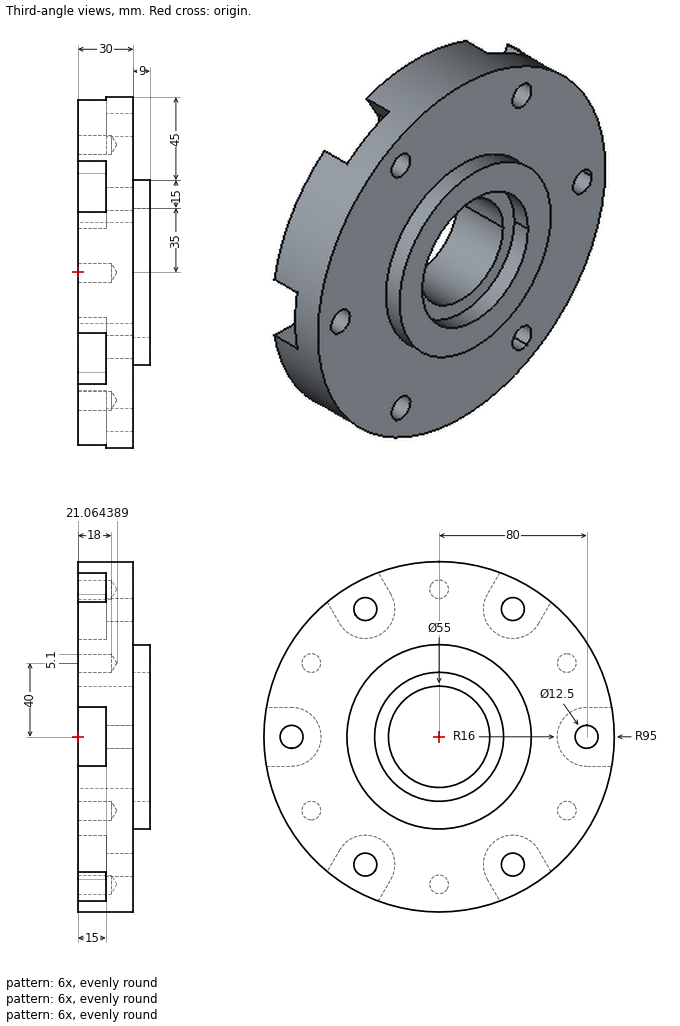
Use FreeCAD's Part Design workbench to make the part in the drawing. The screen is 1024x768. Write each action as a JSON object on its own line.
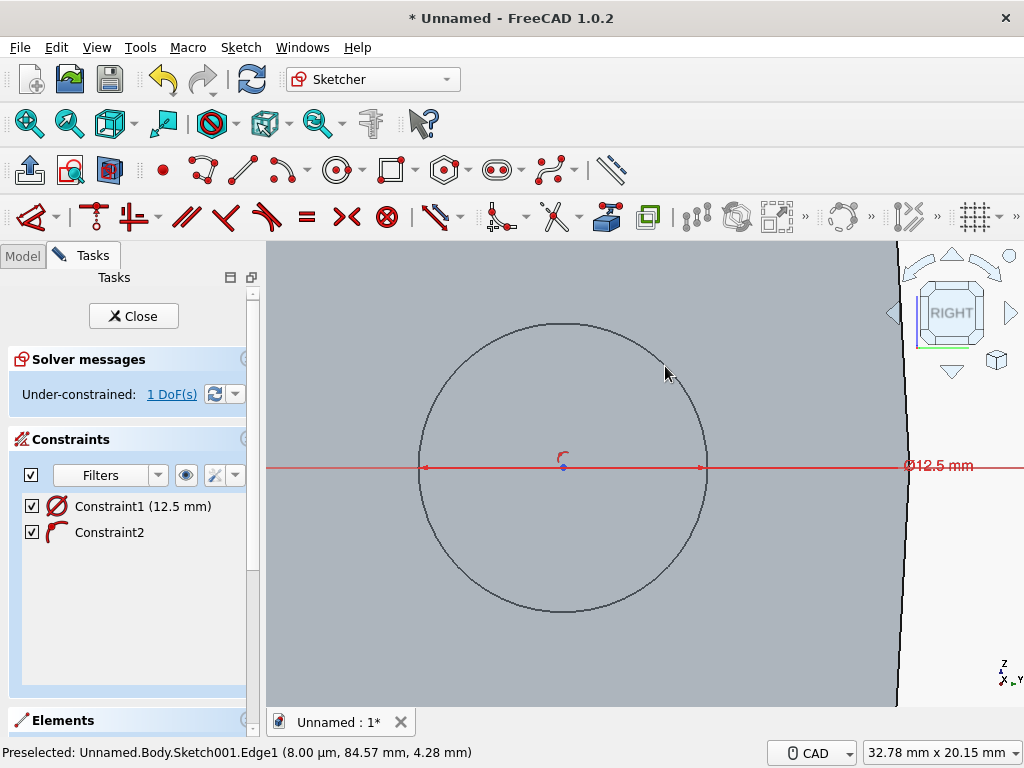
{"action": "key", "text": "d"}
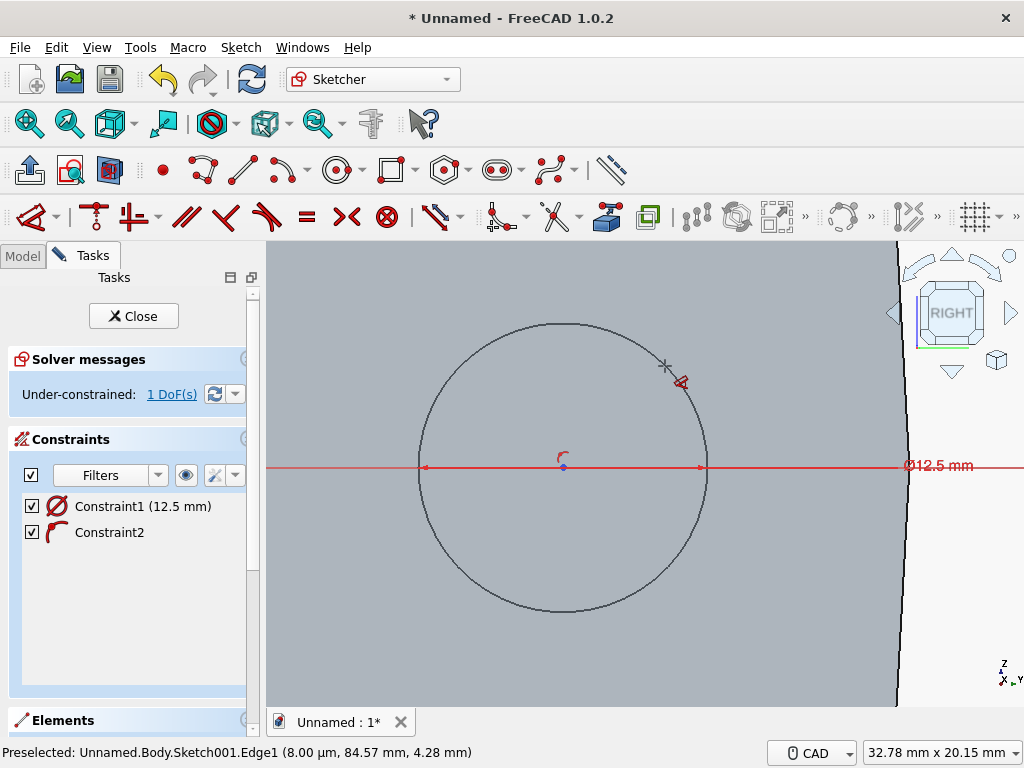
{"action": "left_click", "coordinate": [563, 468]}
{"action": "left_click", "coordinate": [367, 502]}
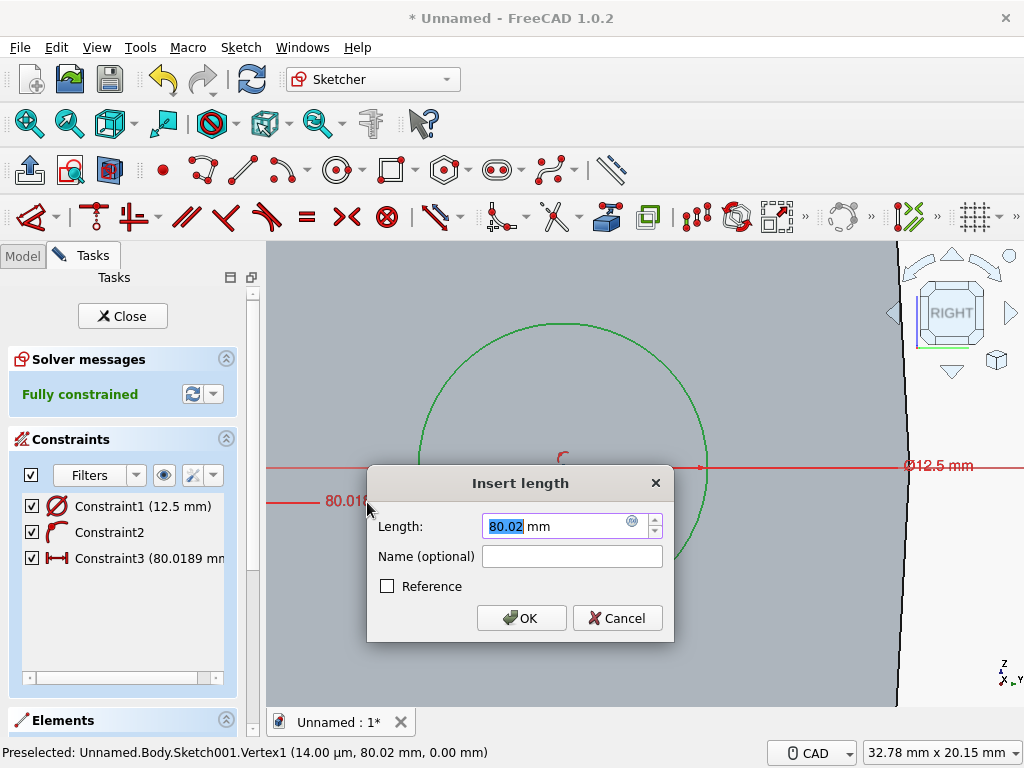
{"action": "type", "text": "80"}
{"action": "key", "text": "Return"}
{"action": "key", "text": "Escape"}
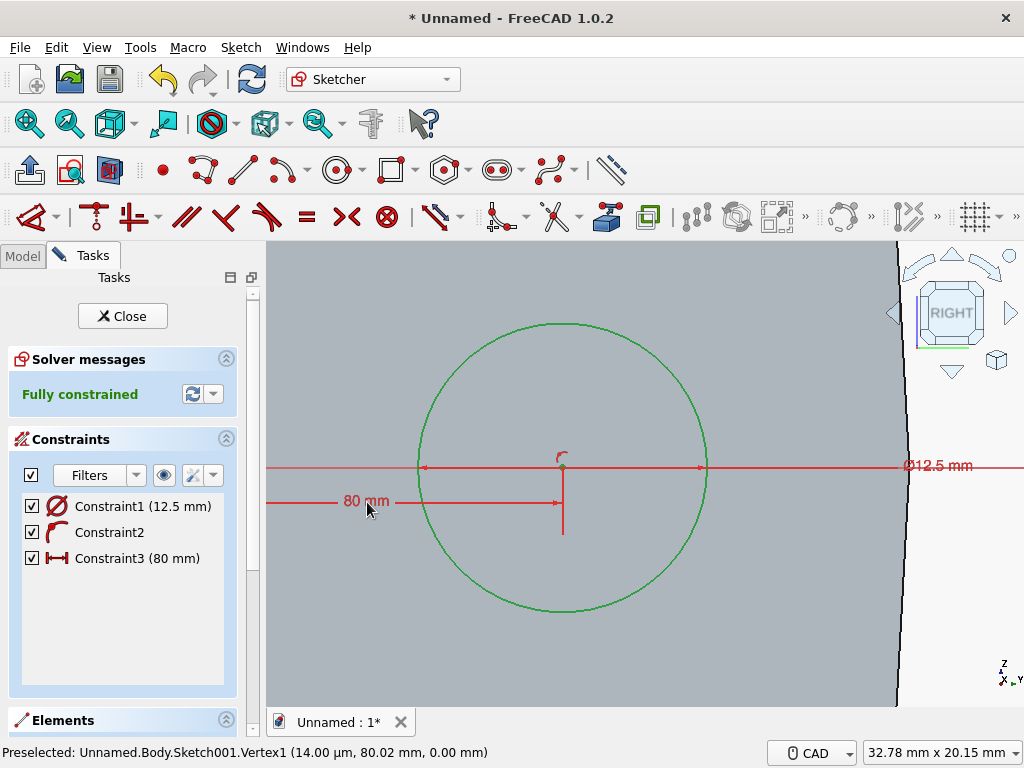
{"action": "left_click", "coordinate": [123, 316]}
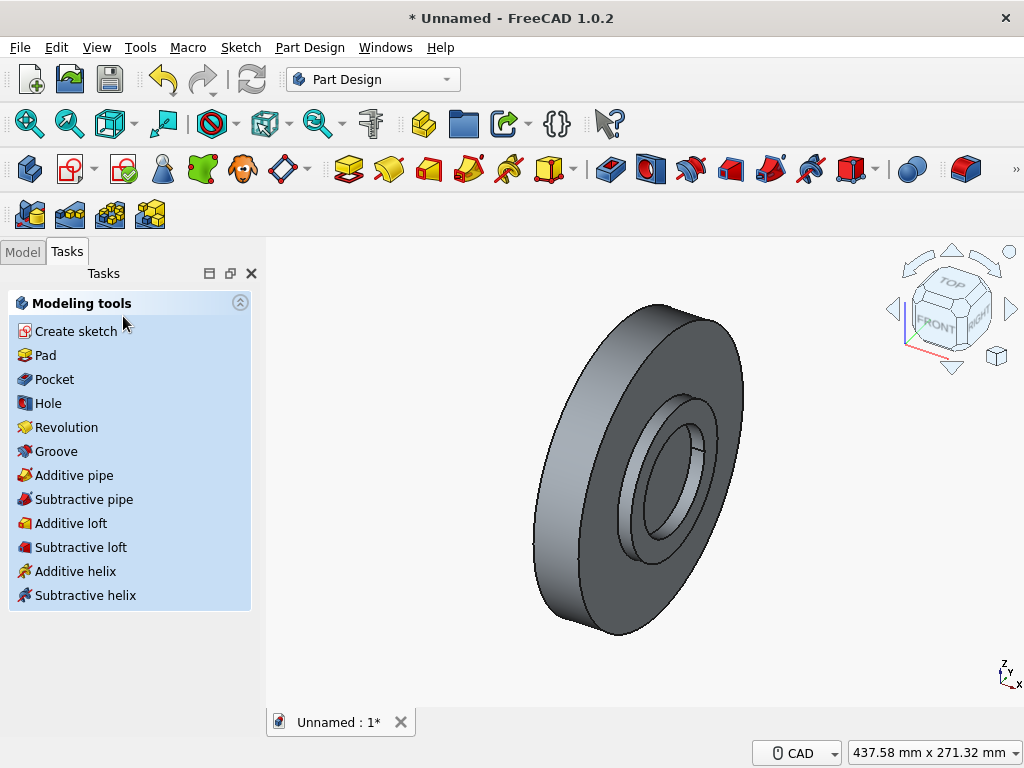
{"action": "left_click", "coordinate": [612, 170]}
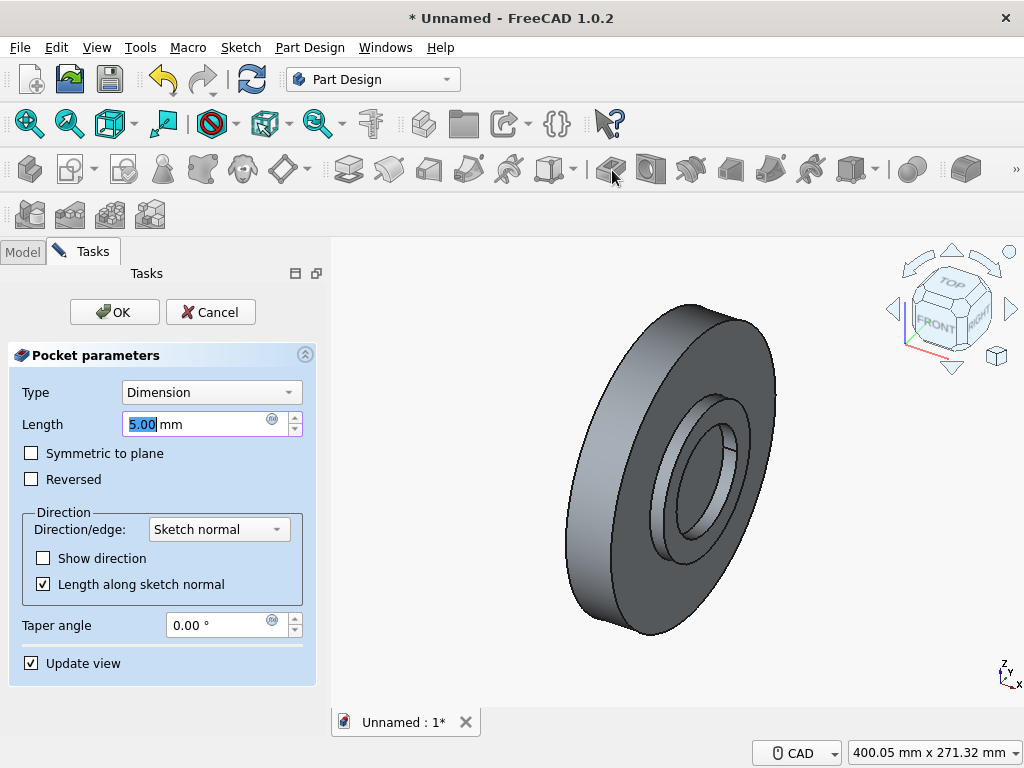
{"action": "left_click", "coordinate": [212, 392]}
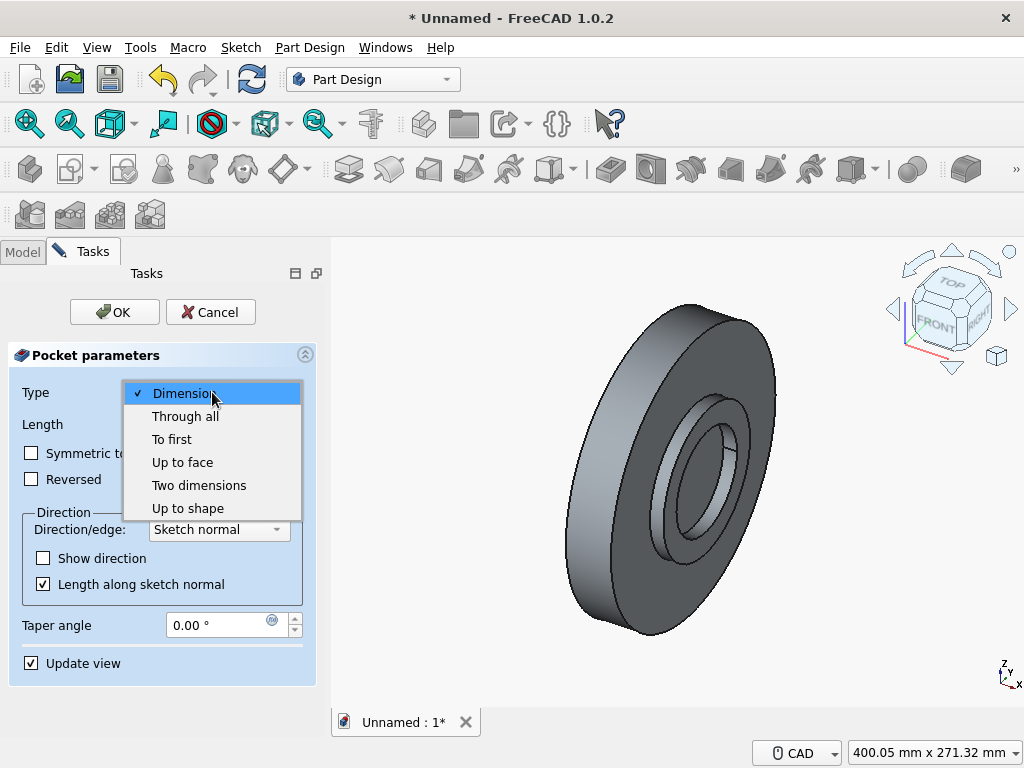
{"action": "left_click", "coordinate": [212, 416]}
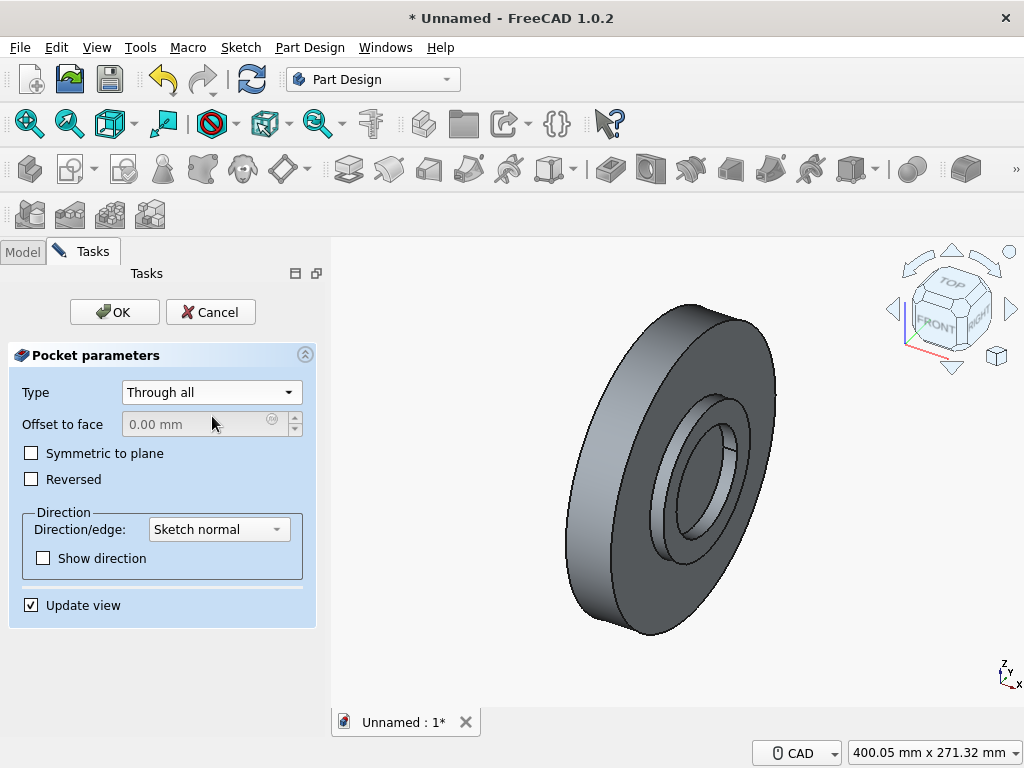
{"action": "left_click", "coordinate": [30, 479]}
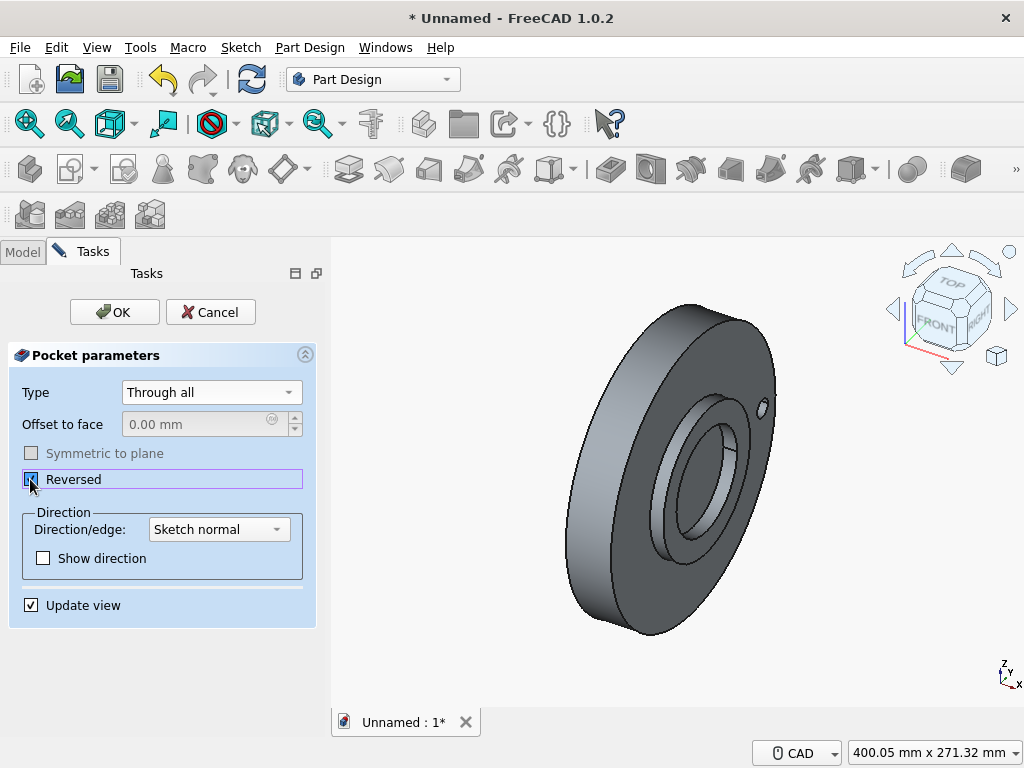
{"action": "left_click", "coordinate": [115, 312]}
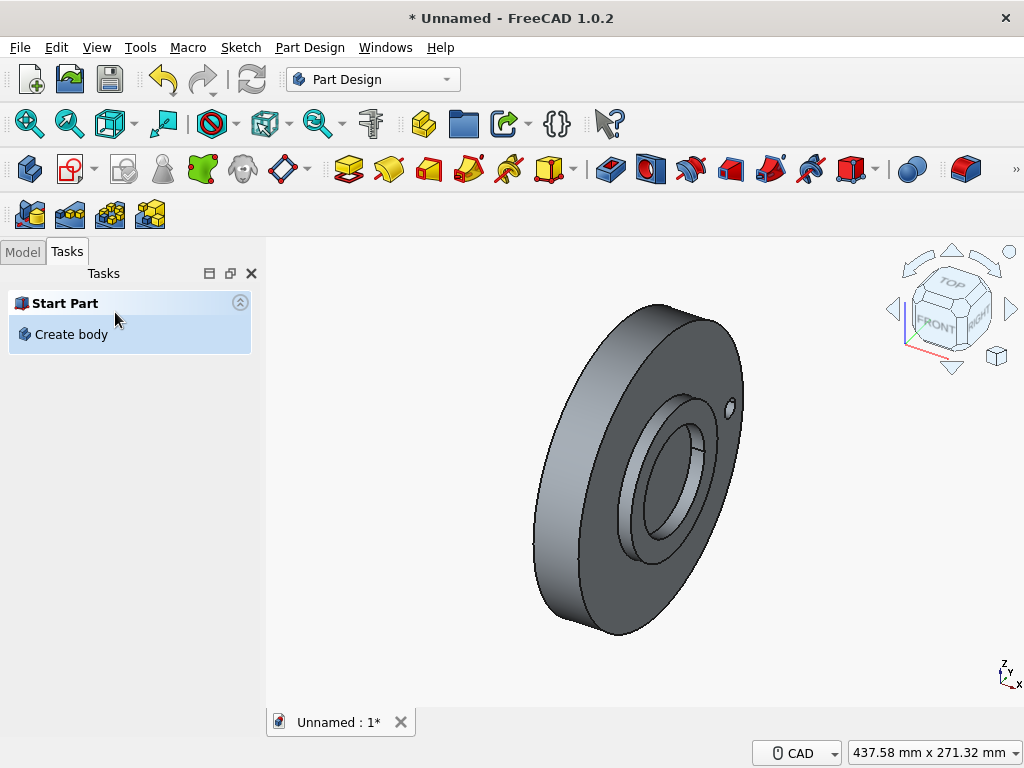
{"action": "left_click", "coordinate": [23, 251]}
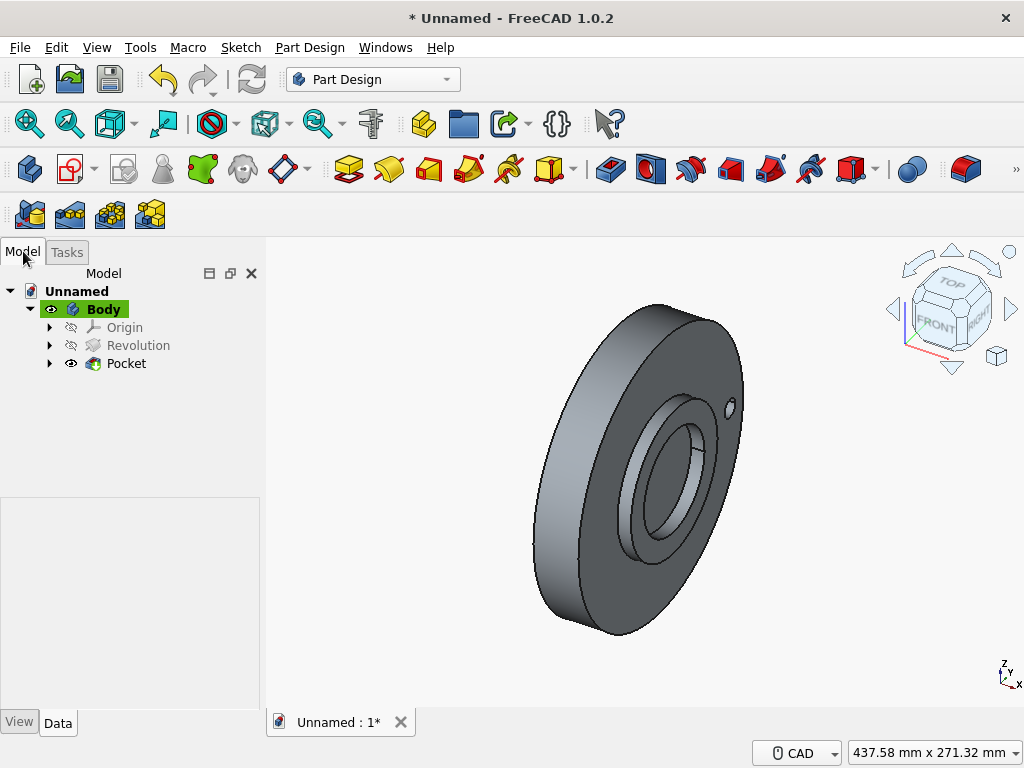
{"action": "left_click", "coordinate": [116, 363]}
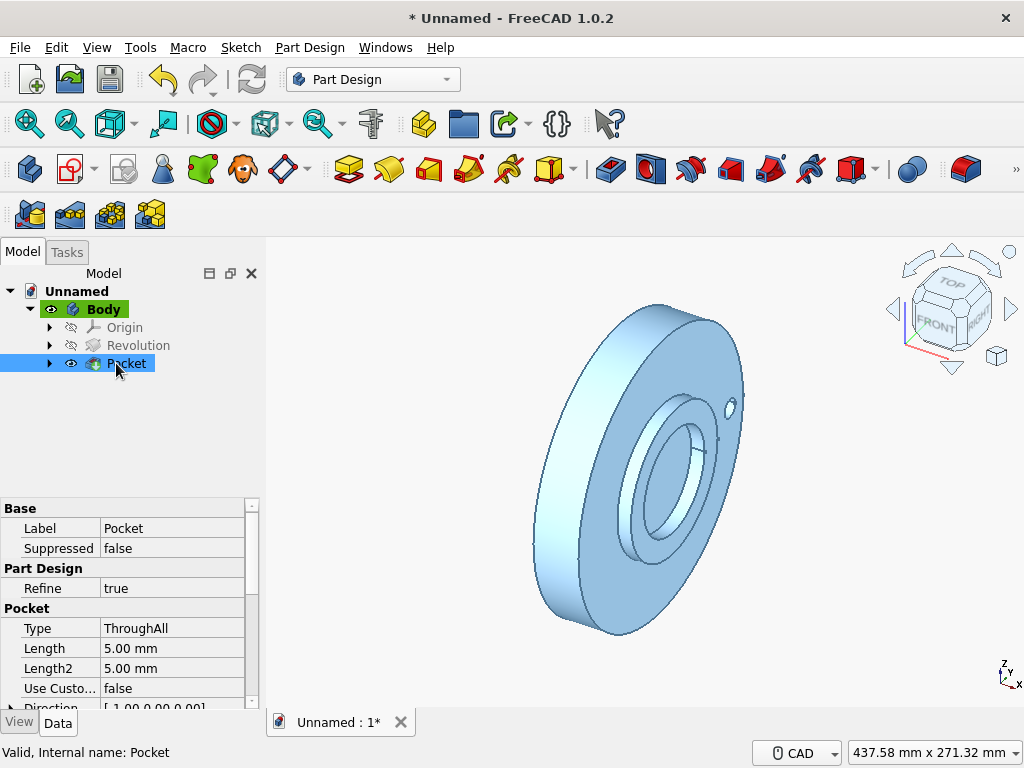
{"action": "left_click", "coordinate": [110, 214]}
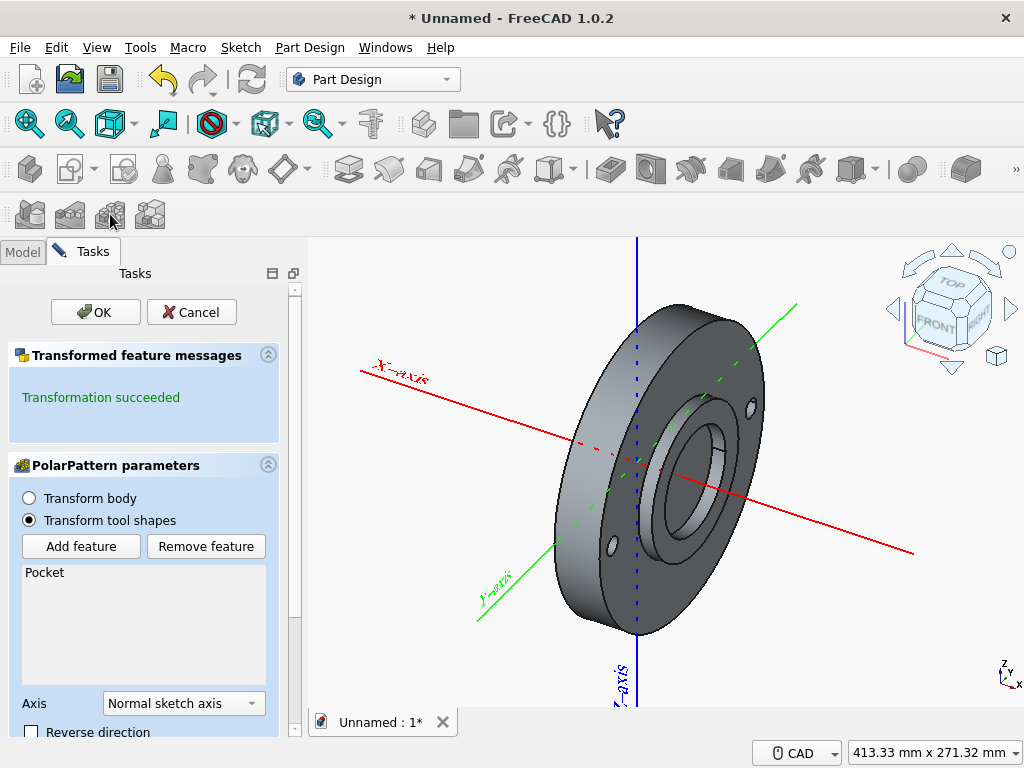
{"action": "left_click", "coordinate": [184, 704]}